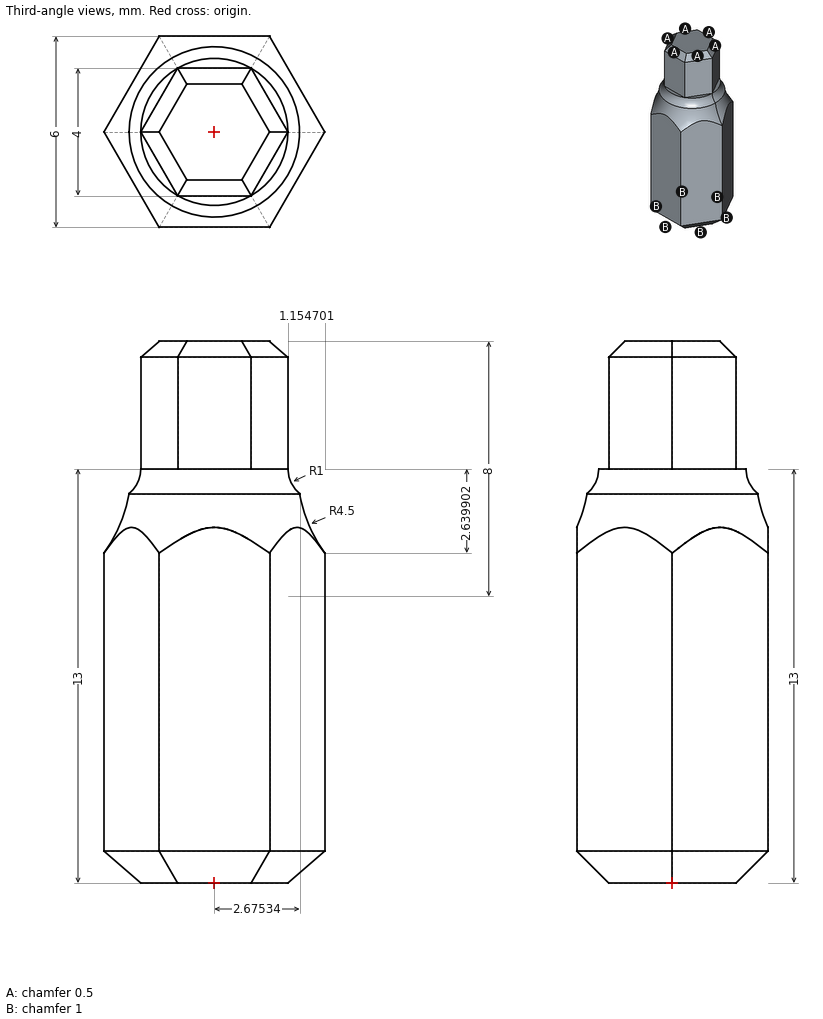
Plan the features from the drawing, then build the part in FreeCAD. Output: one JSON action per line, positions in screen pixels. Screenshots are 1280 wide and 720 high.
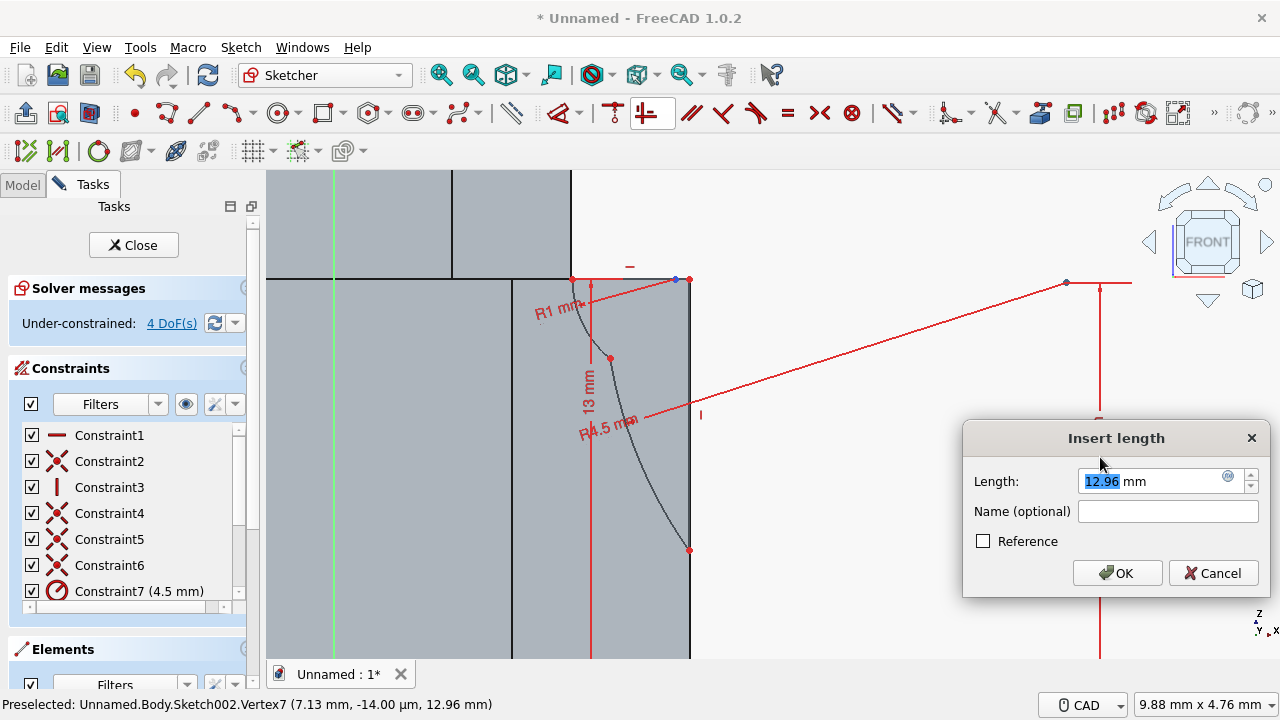
{"action": "type", "text": "13"}
{"action": "key", "text": "Return"}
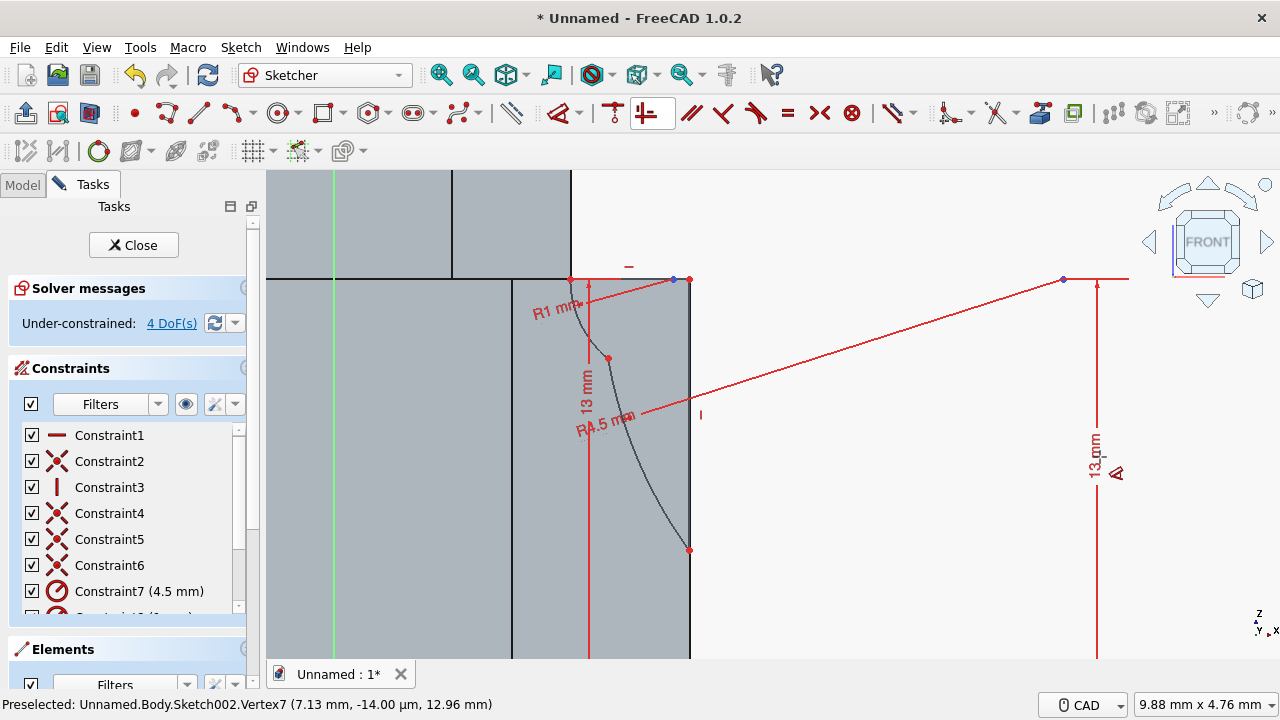
{"action": "left_click", "coordinate": [673, 279]}
{"action": "left_click", "coordinate": [300, 455]}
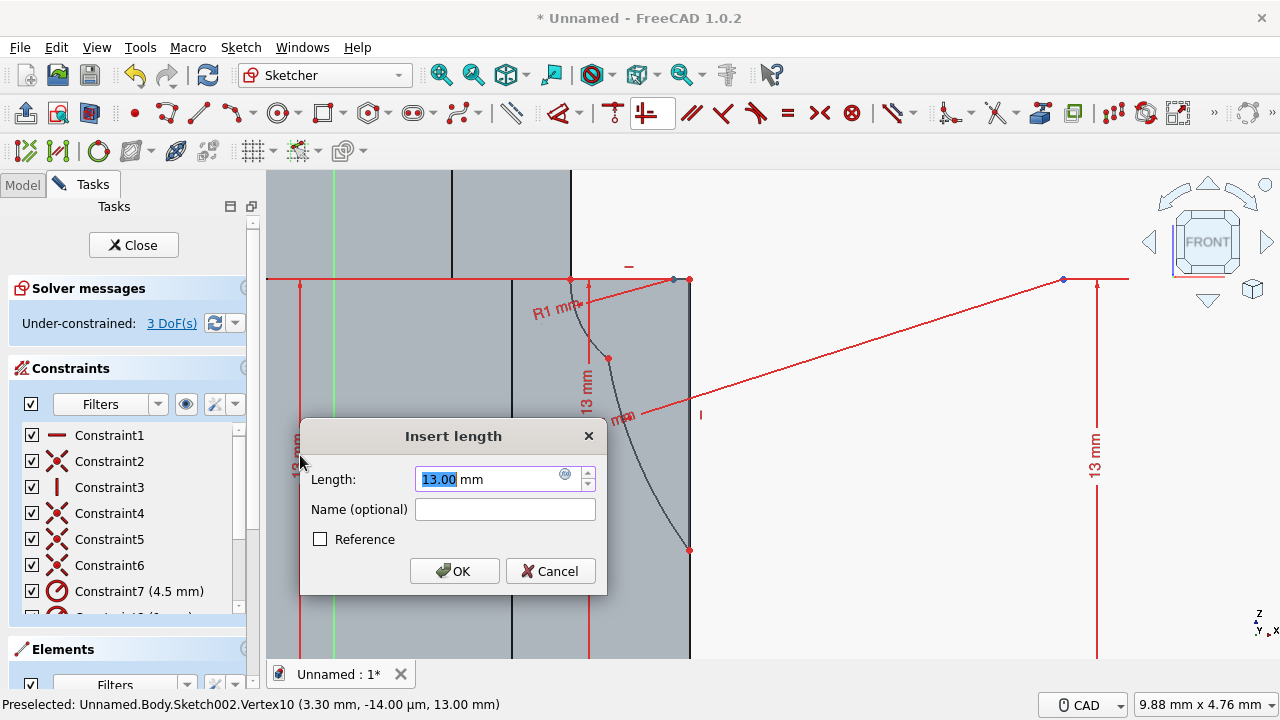
{"action": "type", "text": "13"}
{"action": "key", "text": "Return"}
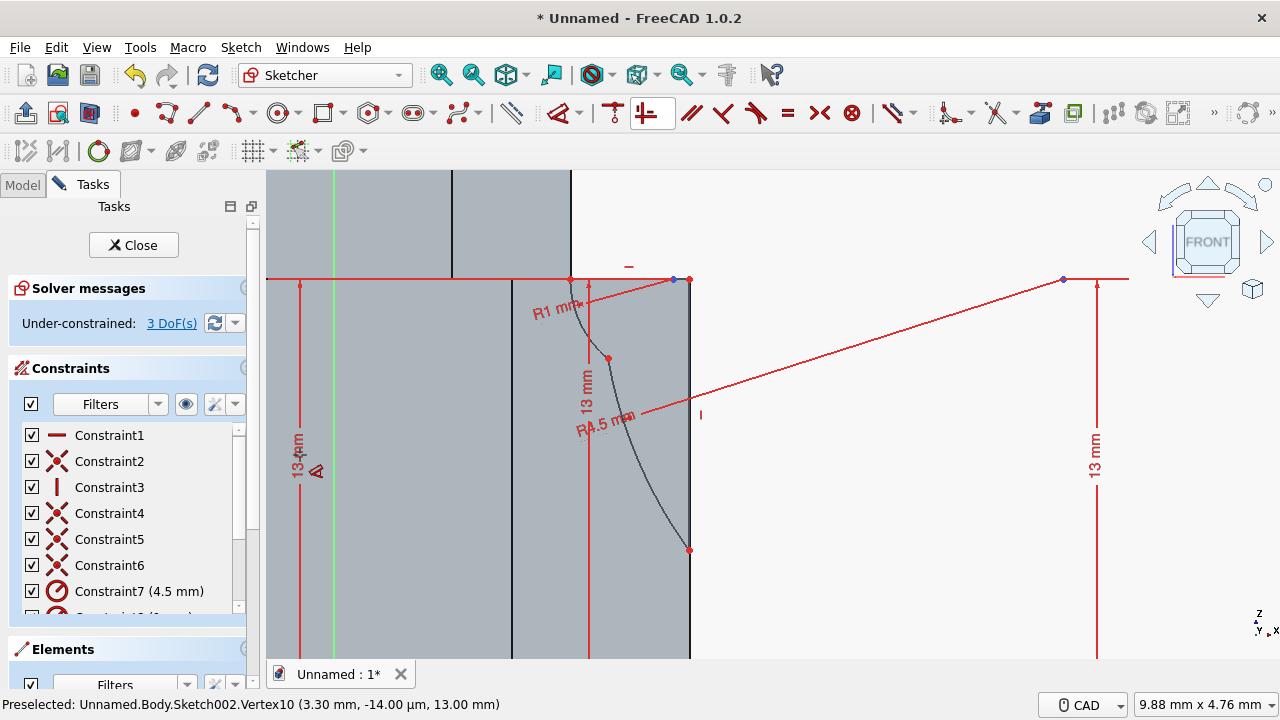
{"action": "left_click", "coordinate": [606, 279]}
{"action": "left_click", "coordinate": [630, 245]}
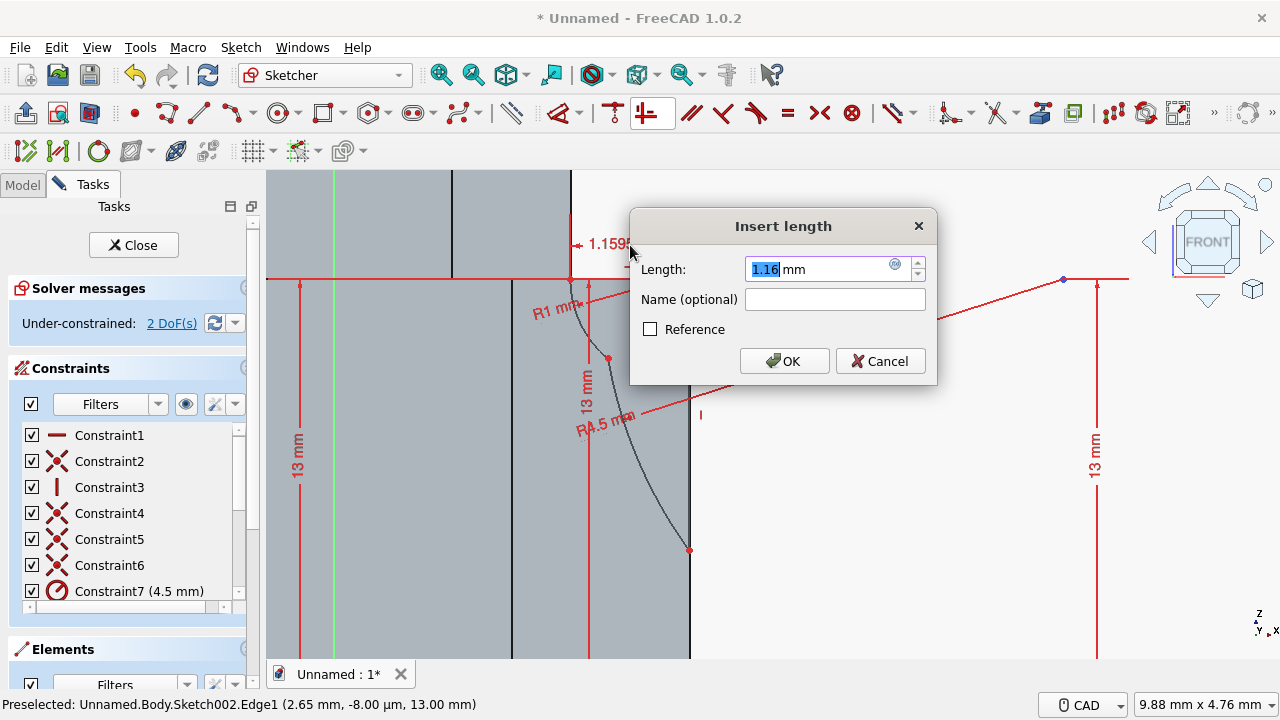
{"action": "type", "text": "1.154701"}
{"action": "key", "text": "Return"}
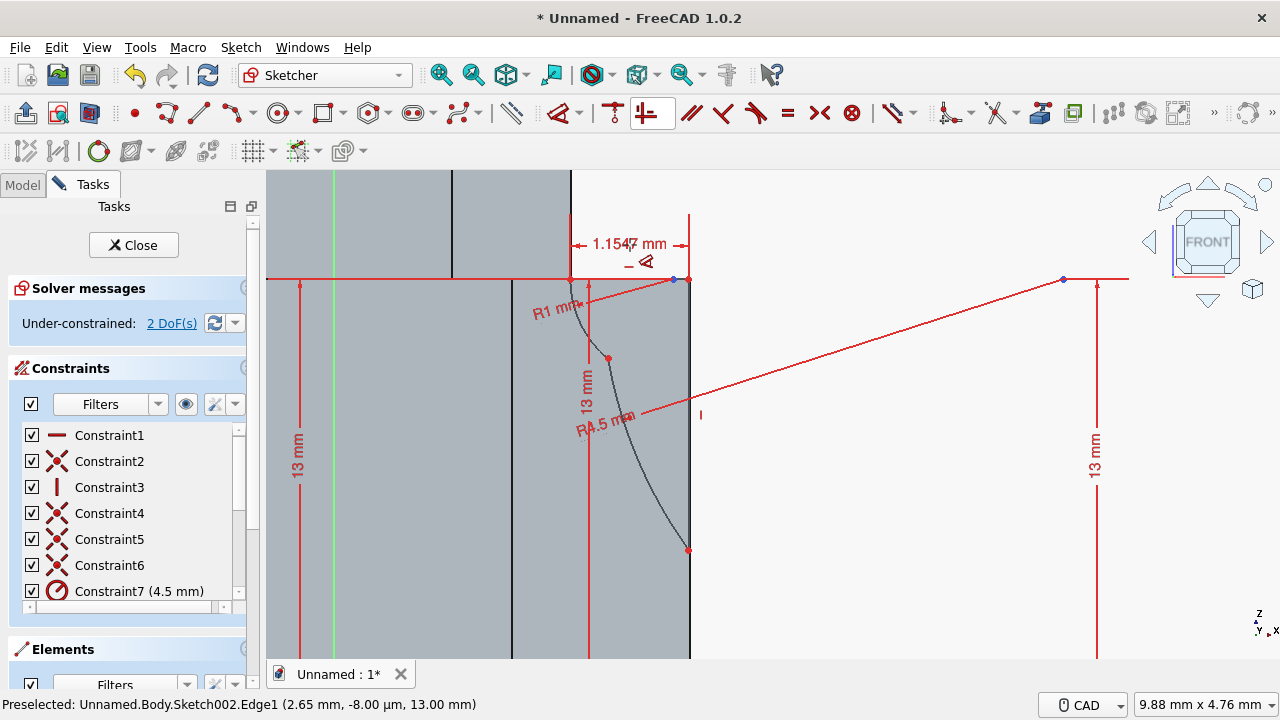
{"action": "left_click", "coordinate": [689, 360]}
{"action": "left_click", "coordinate": [723, 415]}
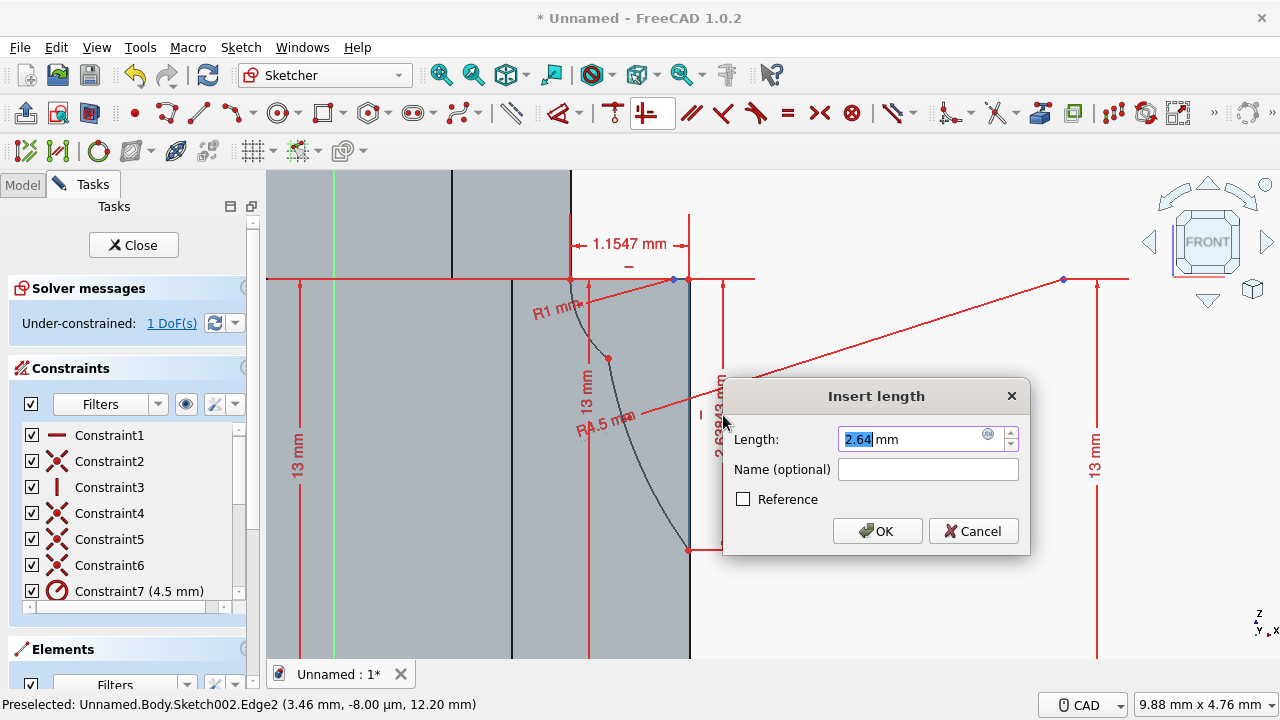
{"action": "type", "text": "2.639902"}
{"action": "key", "text": "Return"}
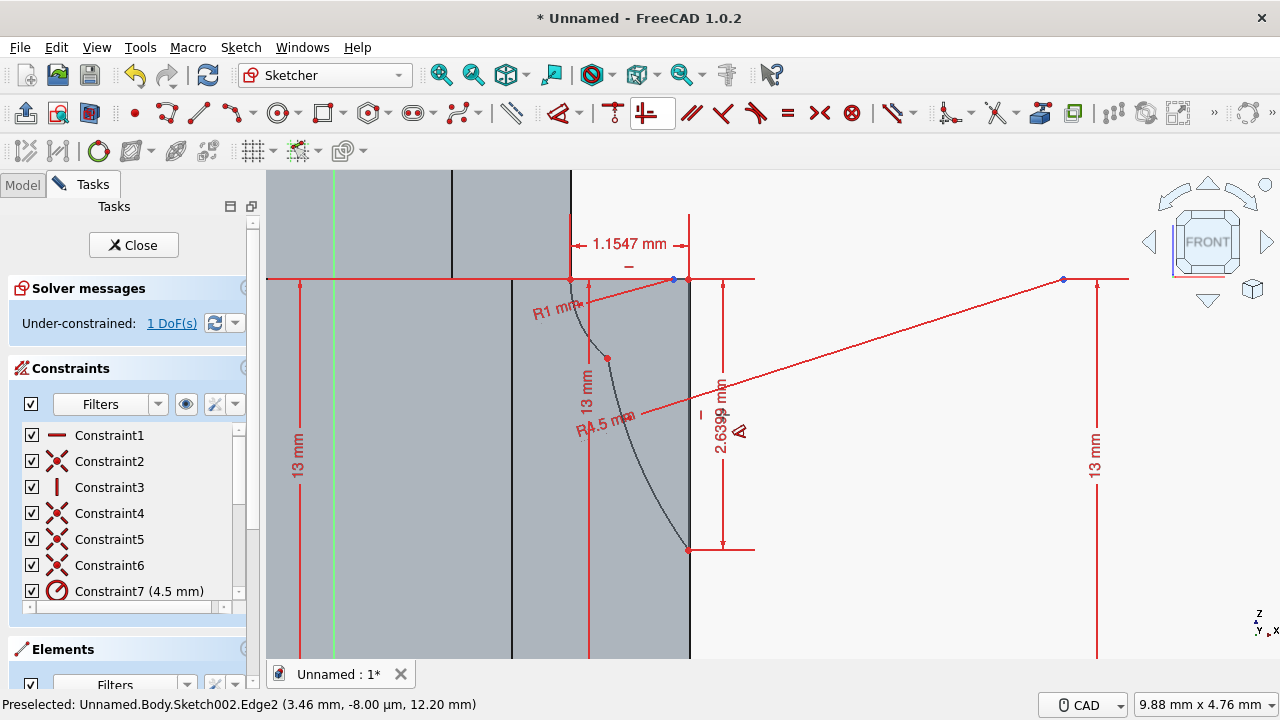
{"action": "left_click", "coordinate": [608, 359]}
{"action": "left_click", "coordinate": [471, 325]}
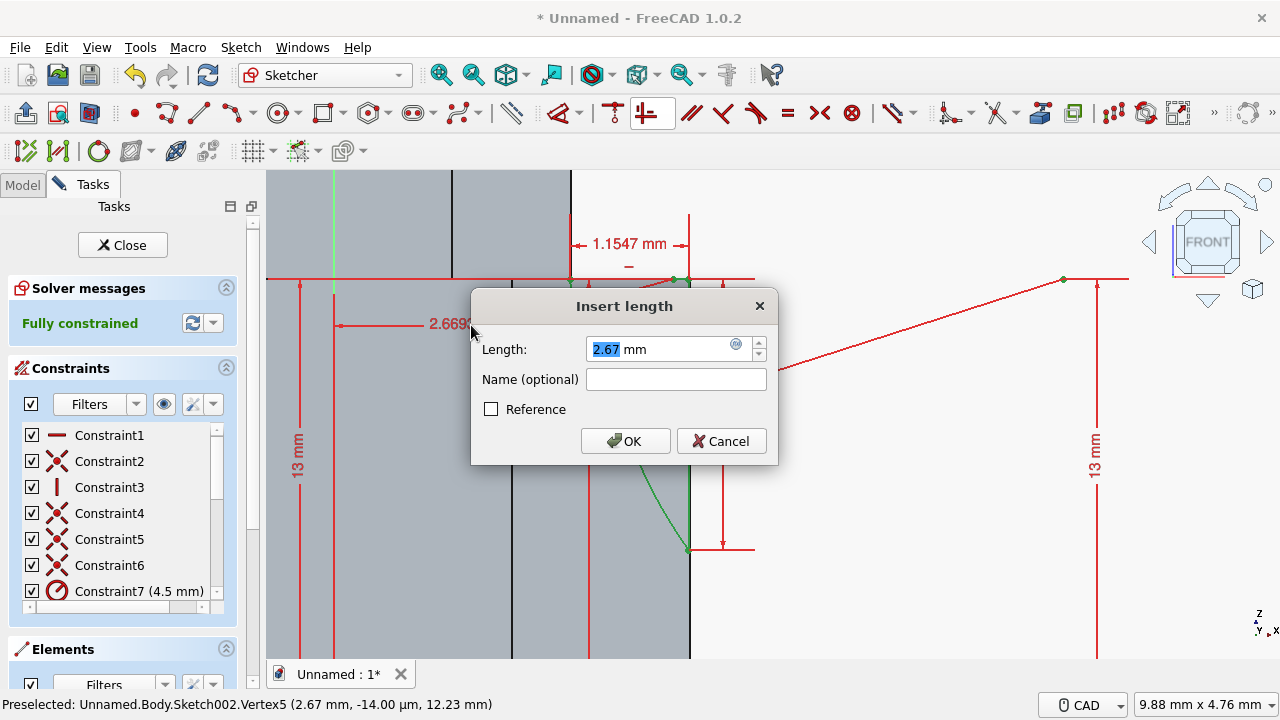
{"action": "type", "text": "2.67534"}
{"action": "key", "text": "Return"}
{"action": "key", "text": "Escape"}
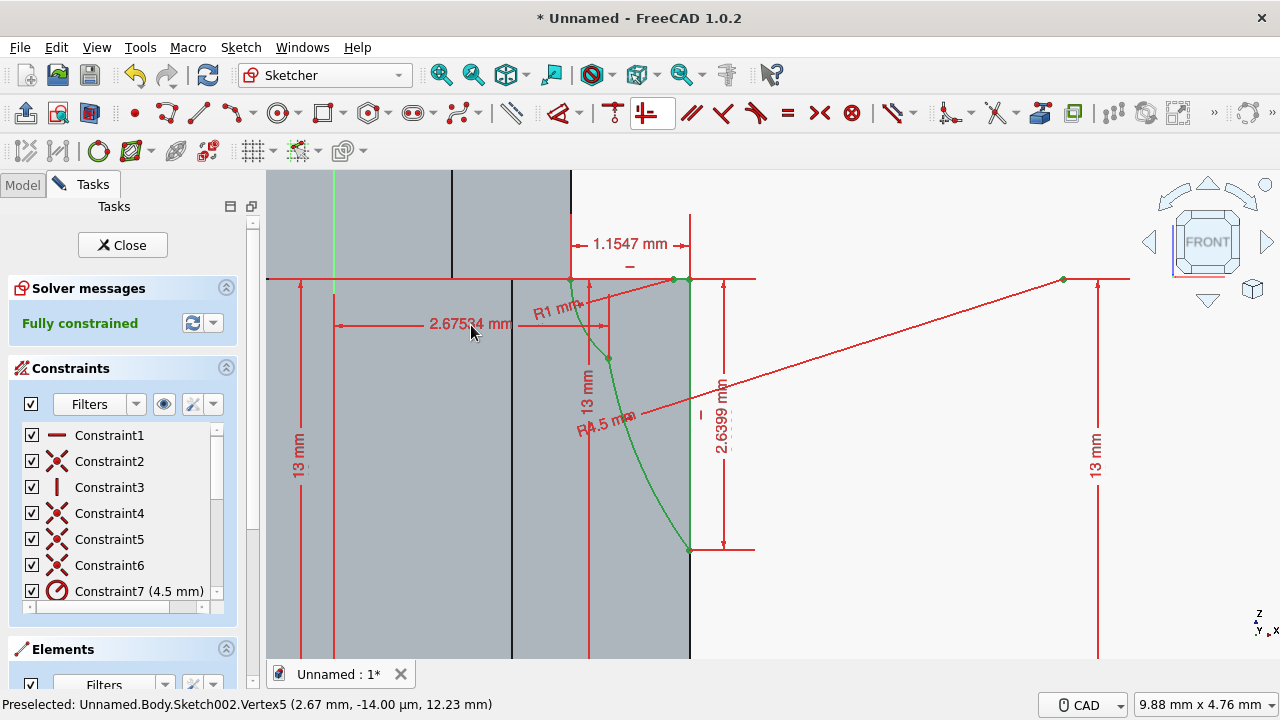
{"action": "left_click", "coordinate": [123, 245]}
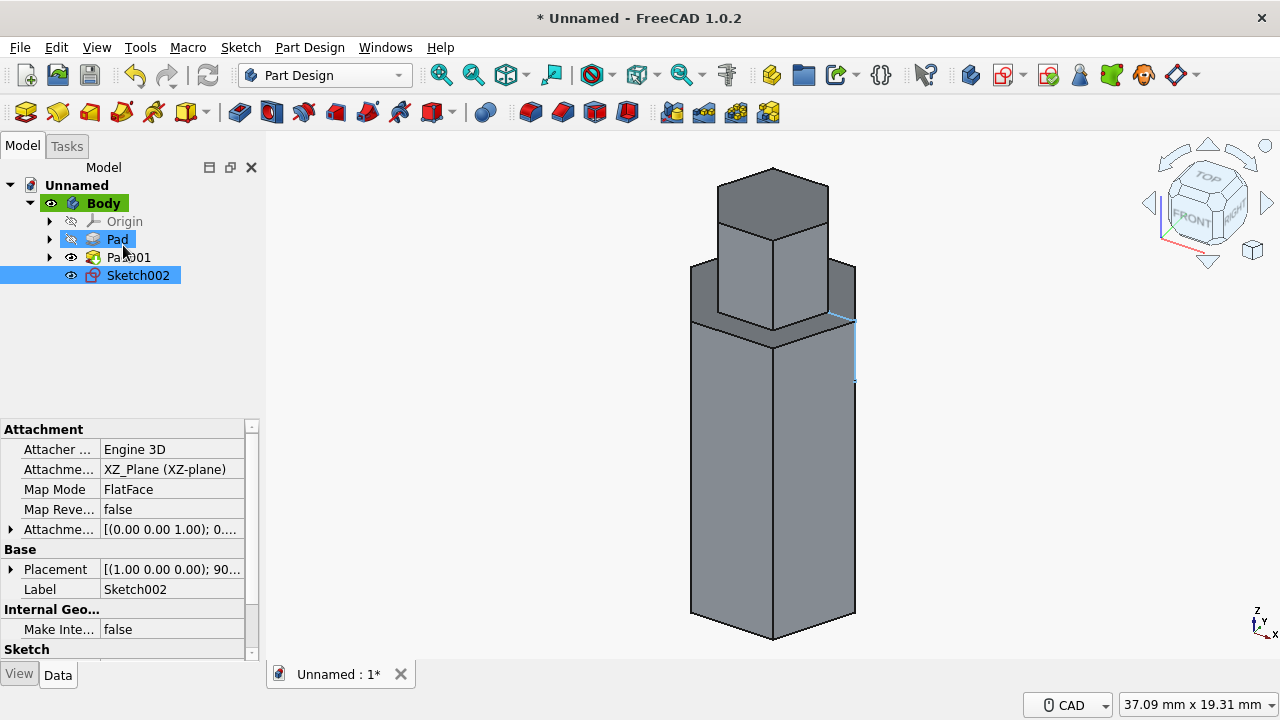
{"action": "left_click", "coordinate": [304, 112]}